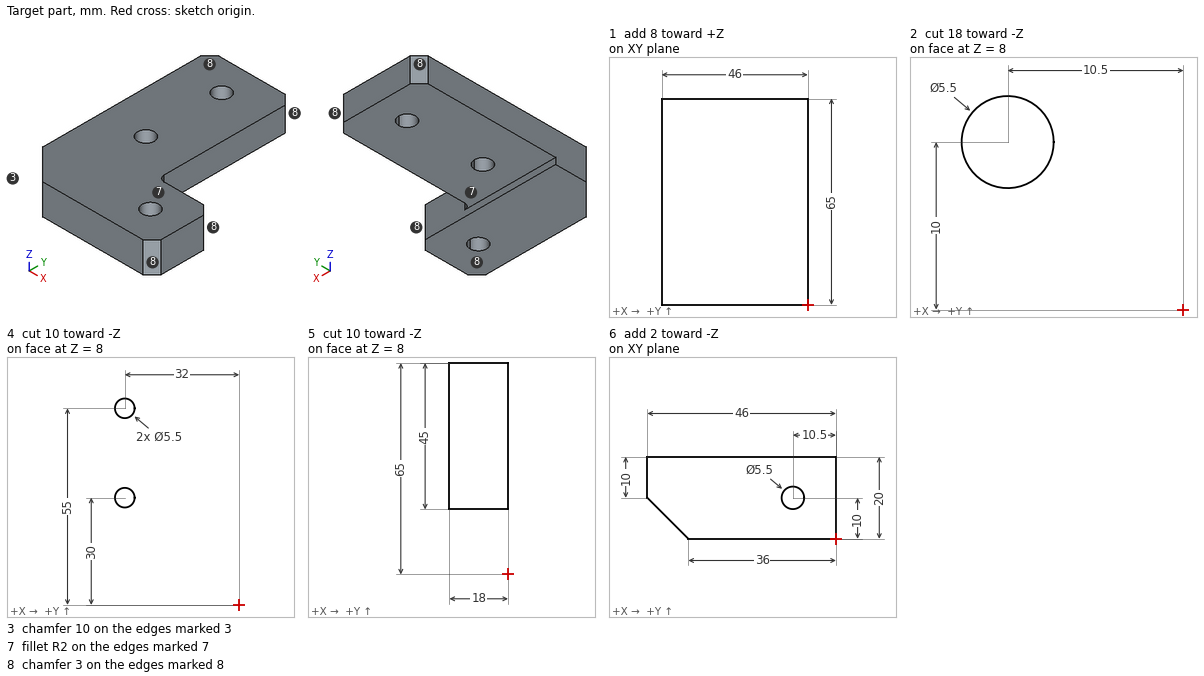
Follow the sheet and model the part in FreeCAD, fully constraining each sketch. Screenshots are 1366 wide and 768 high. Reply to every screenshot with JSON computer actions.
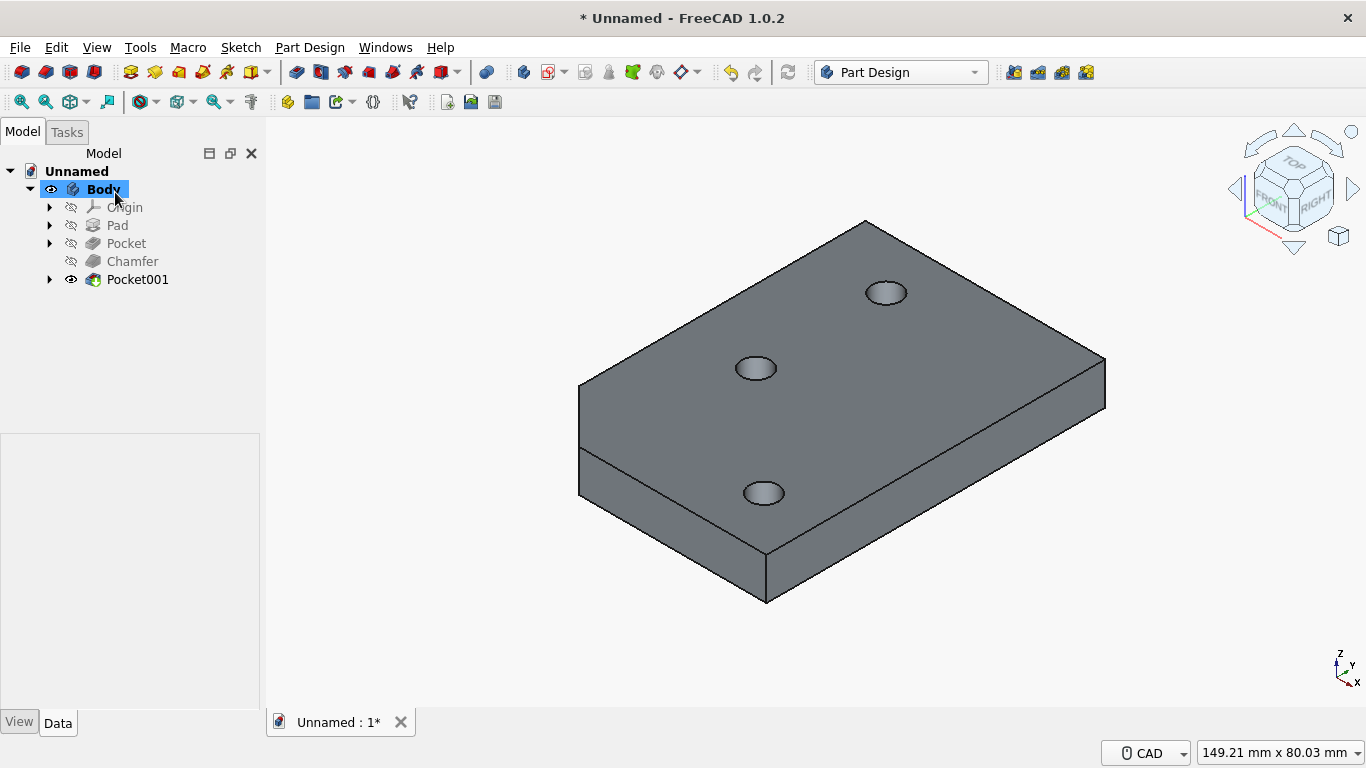
{"action": "left_click", "coordinate": [899, 379]}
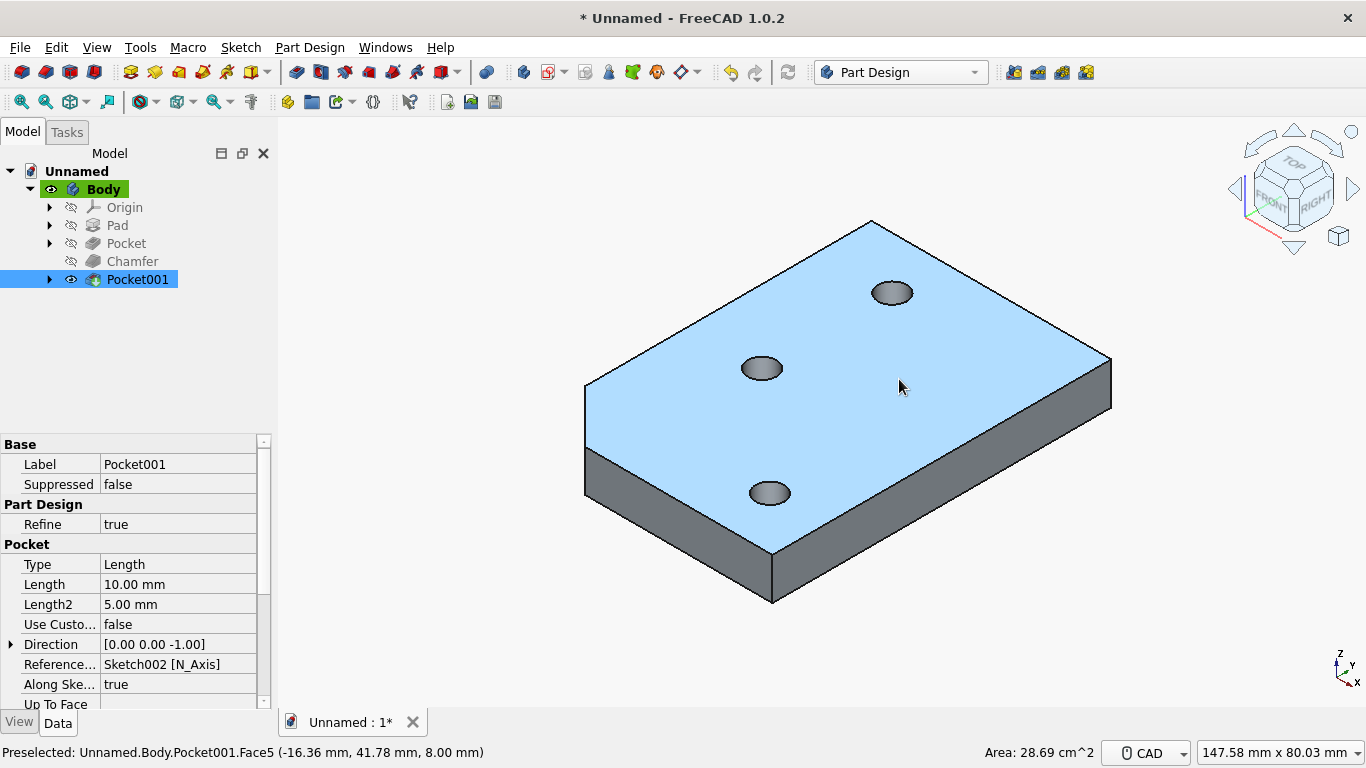
{"action": "left_click", "coordinate": [548, 72]}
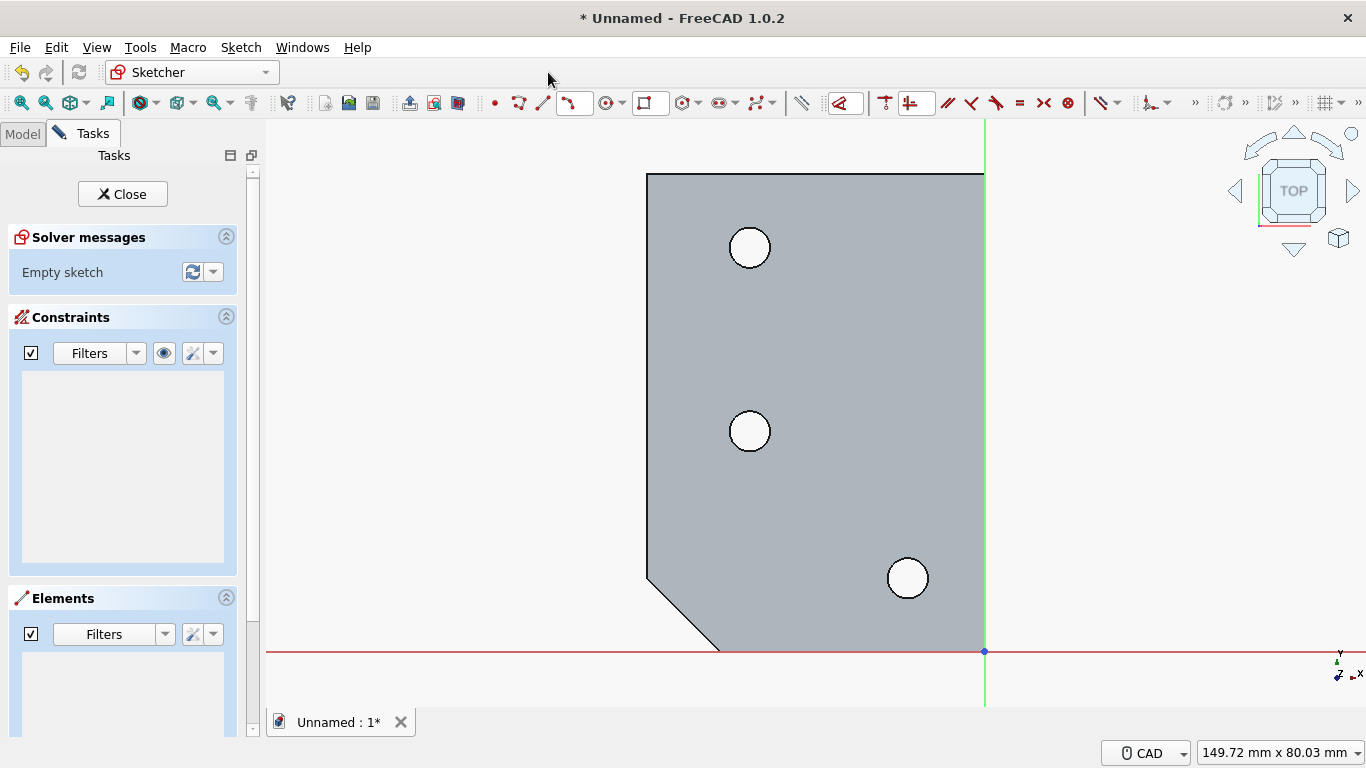
{"action": "left_click", "coordinate": [644, 104]}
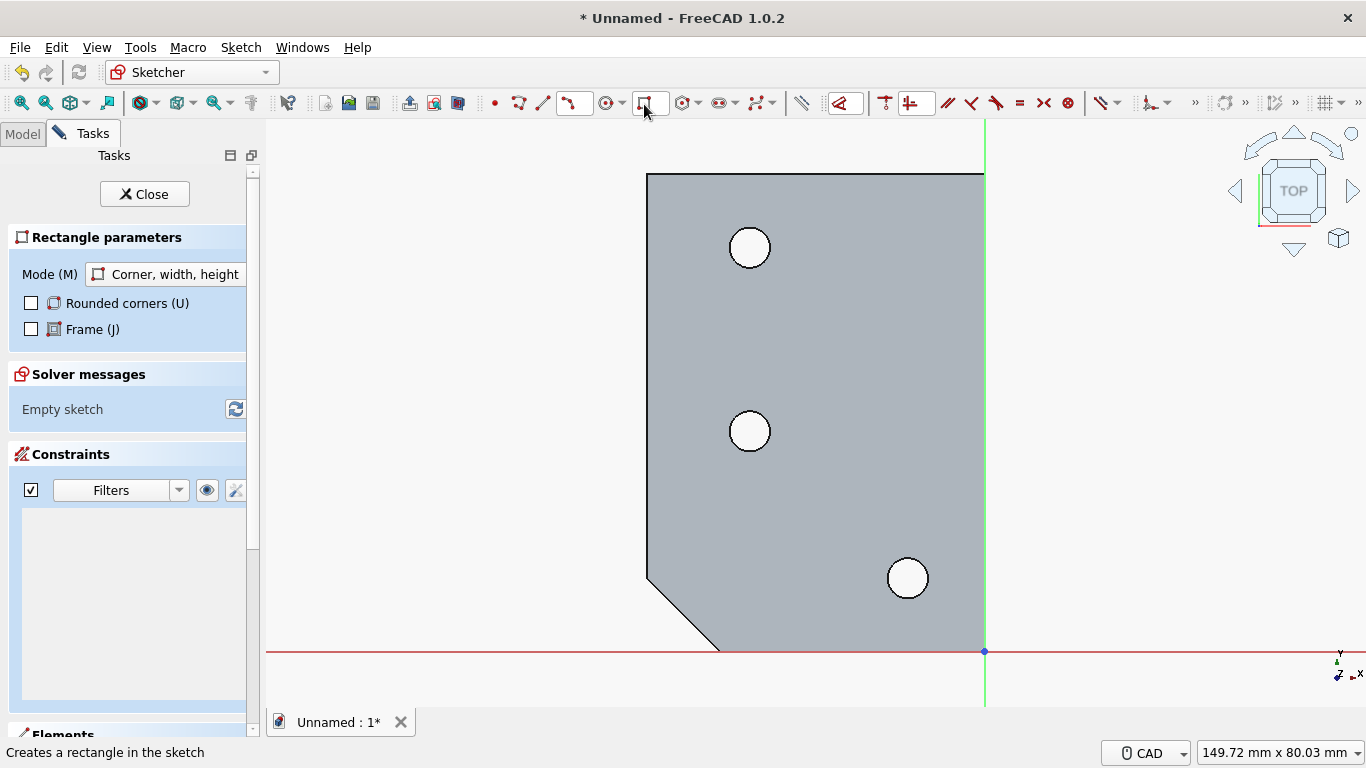
{"action": "left_click", "coordinate": [853, 174]}
{"action": "left_click", "coordinate": [985, 505]}
{"action": "key", "text": "Escape"}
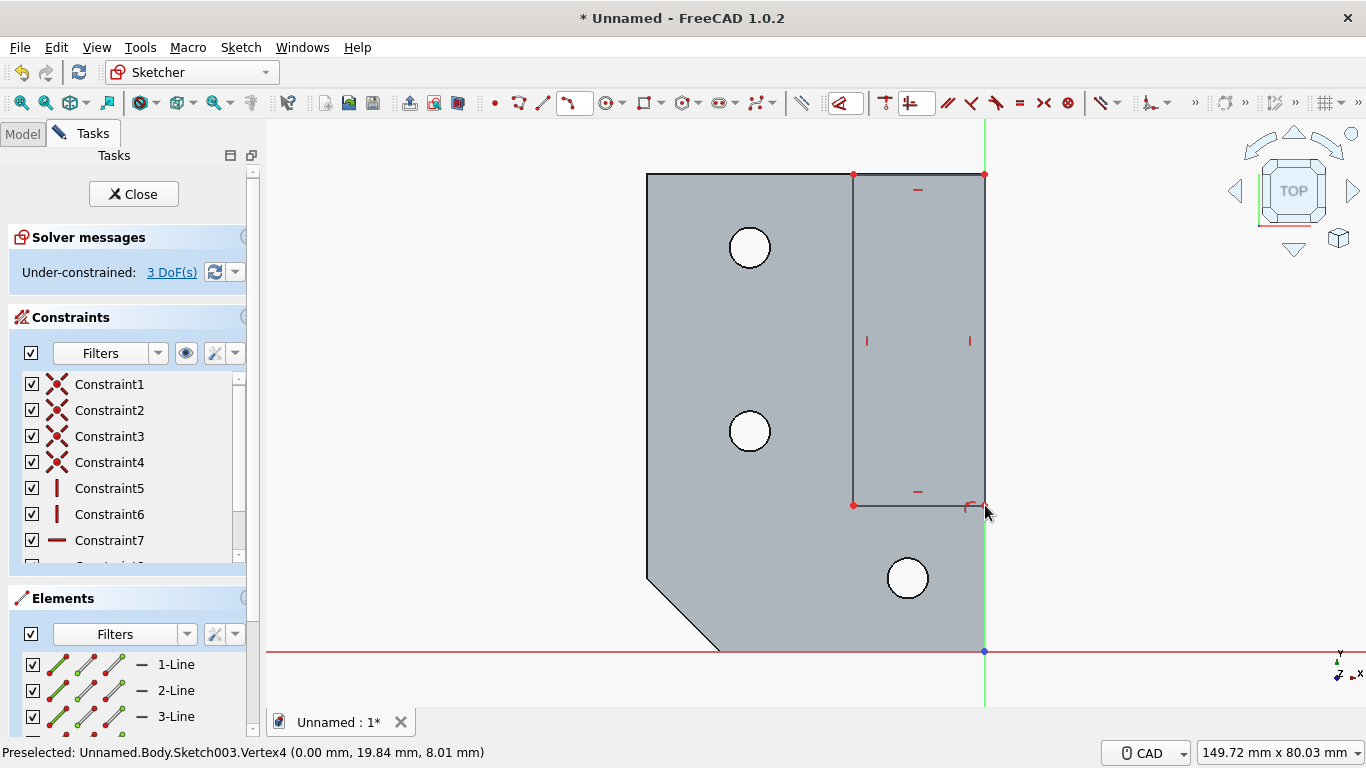
{"action": "left_click", "coordinate": [853, 274]}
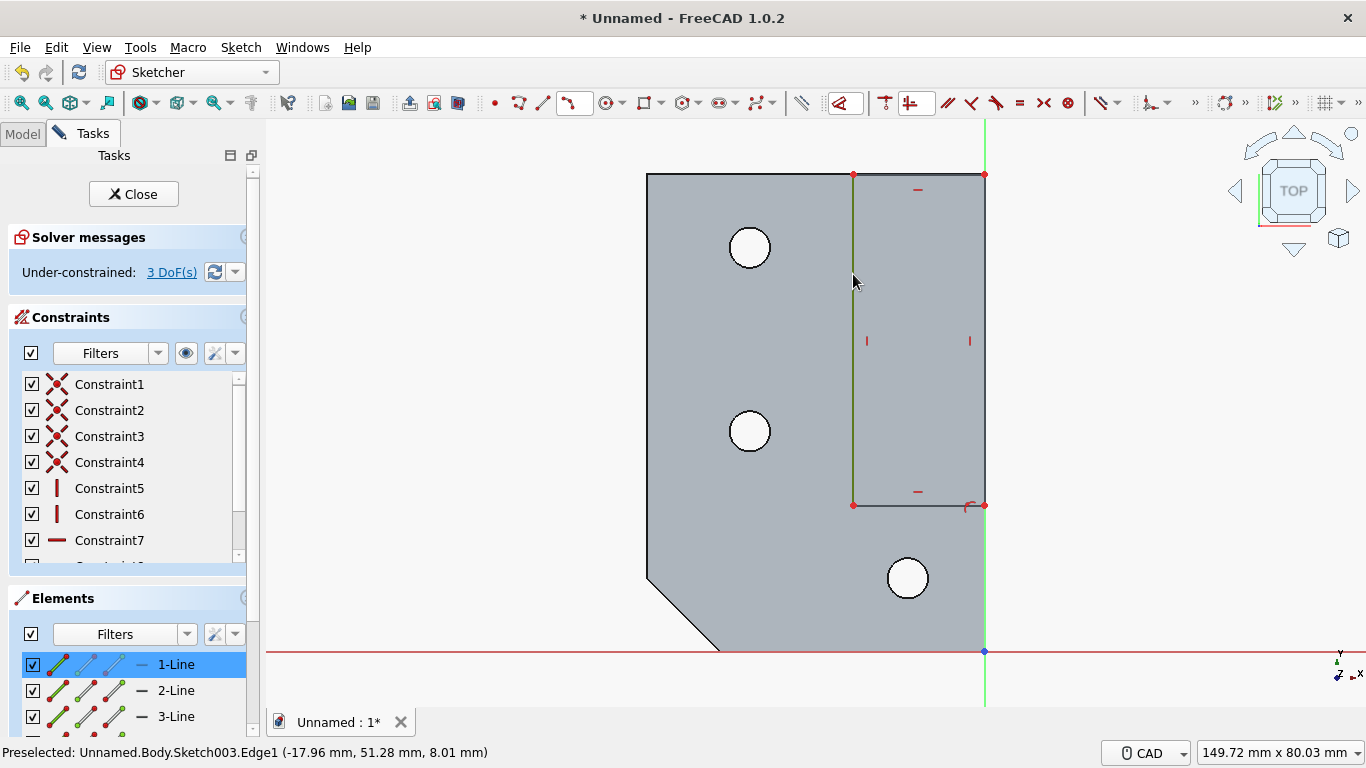
{"action": "key", "text": "i"}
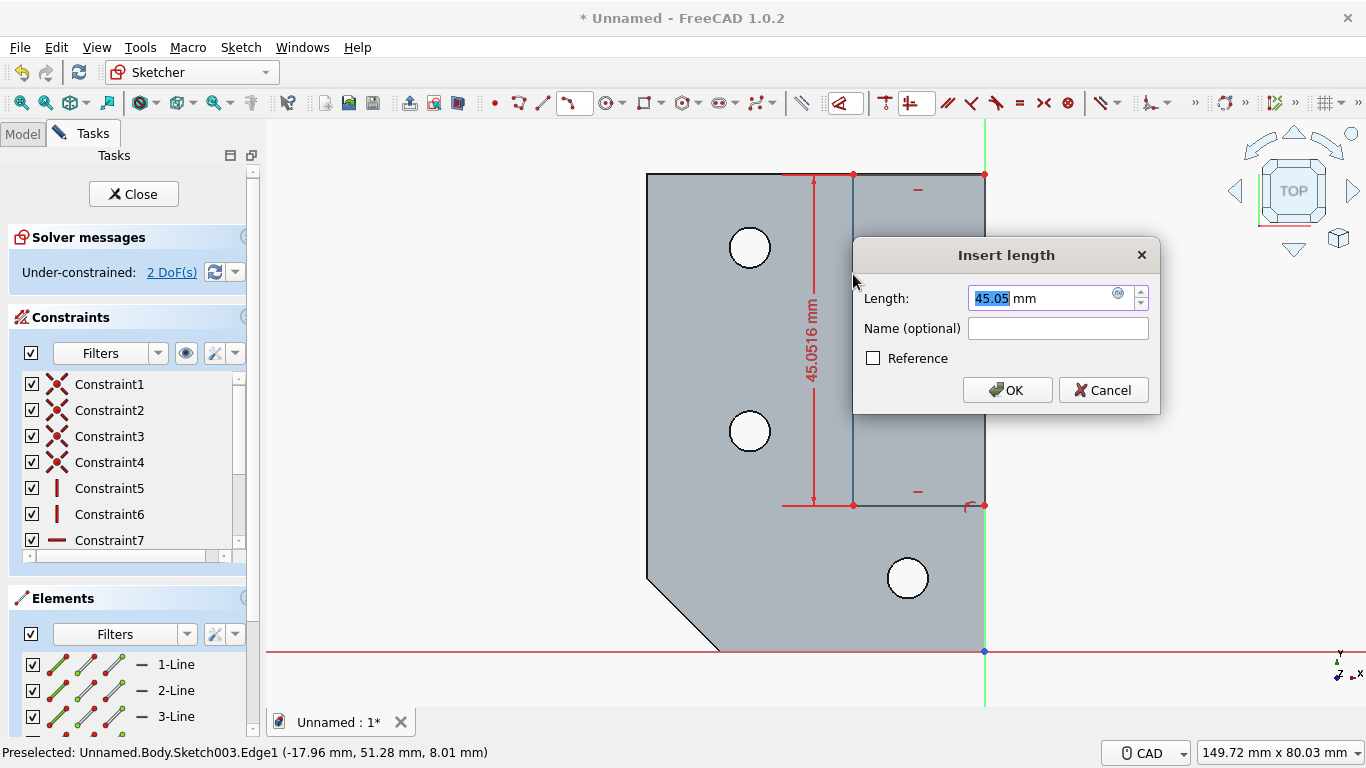
{"action": "type", "text": "45"}
{"action": "key", "text": "Return"}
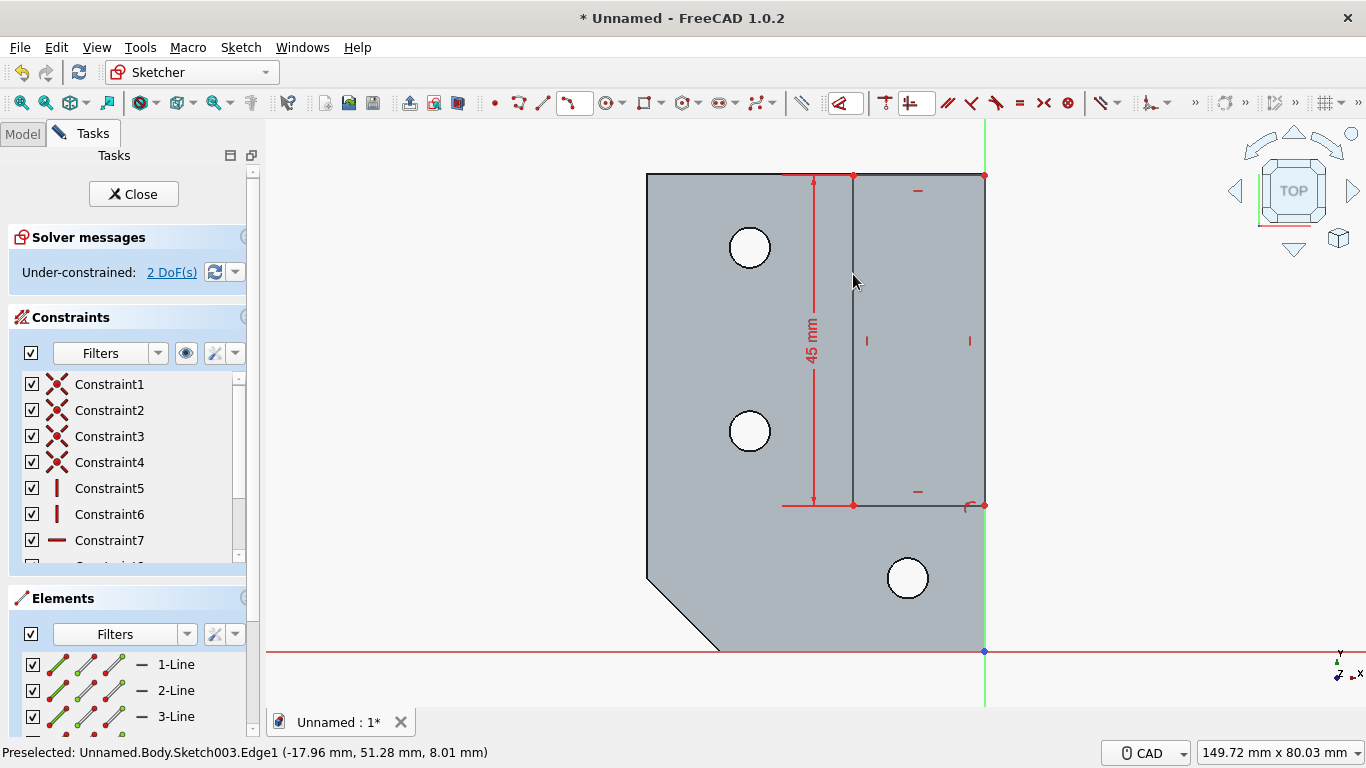
{"action": "left_click", "coordinate": [893, 506]}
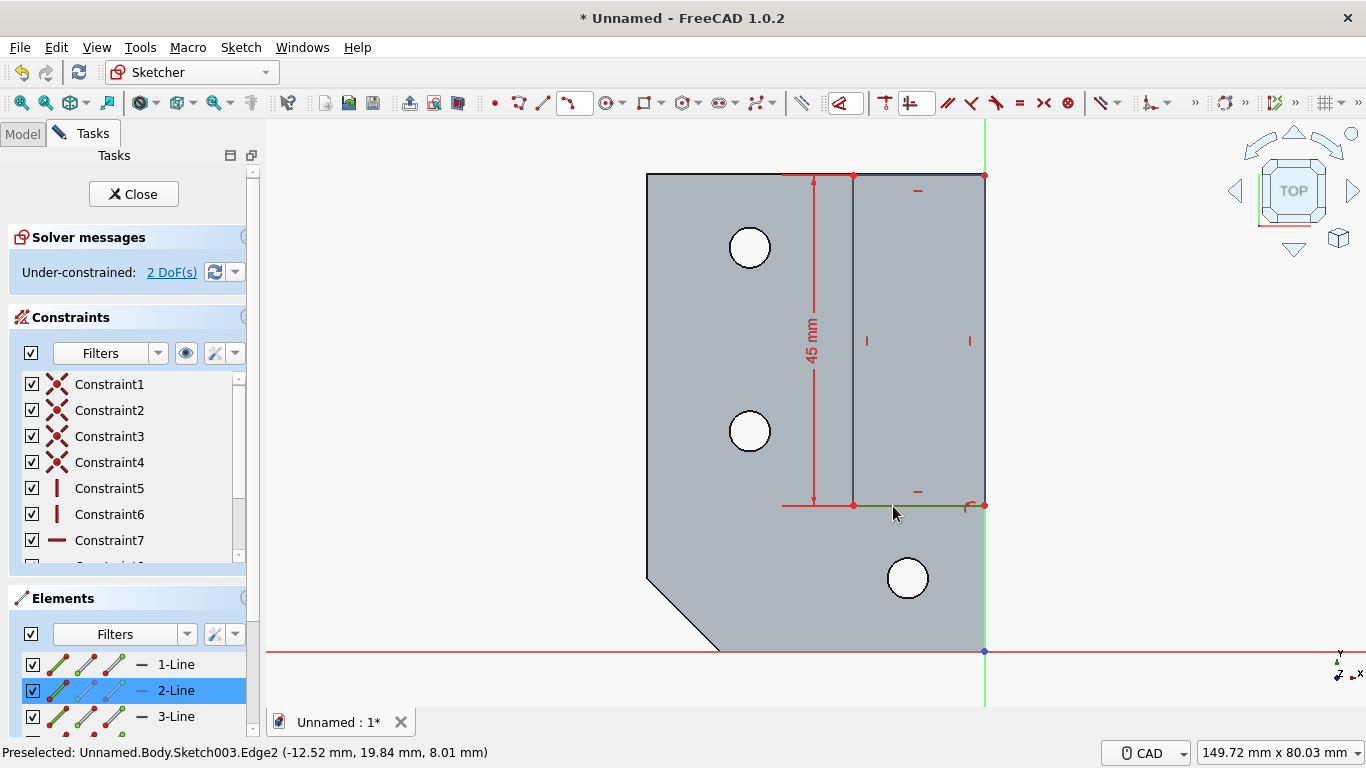
{"action": "key", "text": "l"}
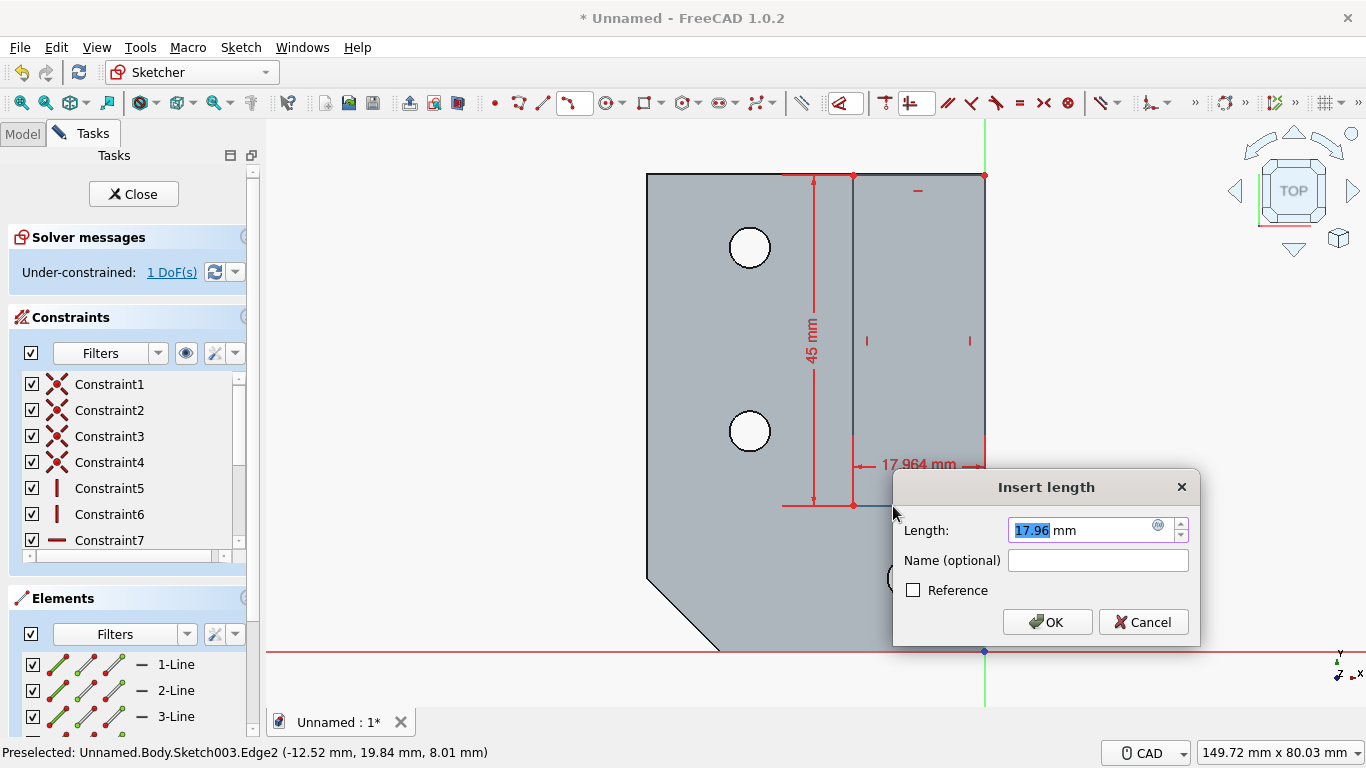
{"action": "type", "text": "18"}
{"action": "key", "text": "Return"}